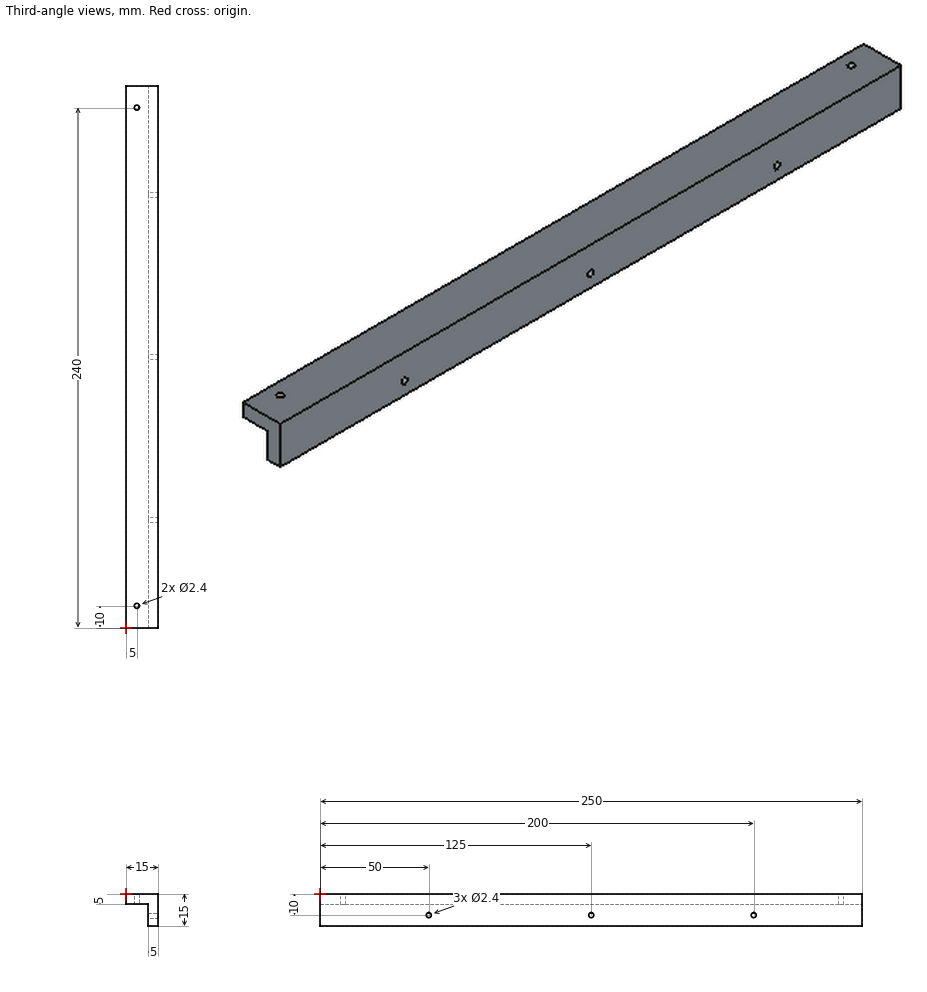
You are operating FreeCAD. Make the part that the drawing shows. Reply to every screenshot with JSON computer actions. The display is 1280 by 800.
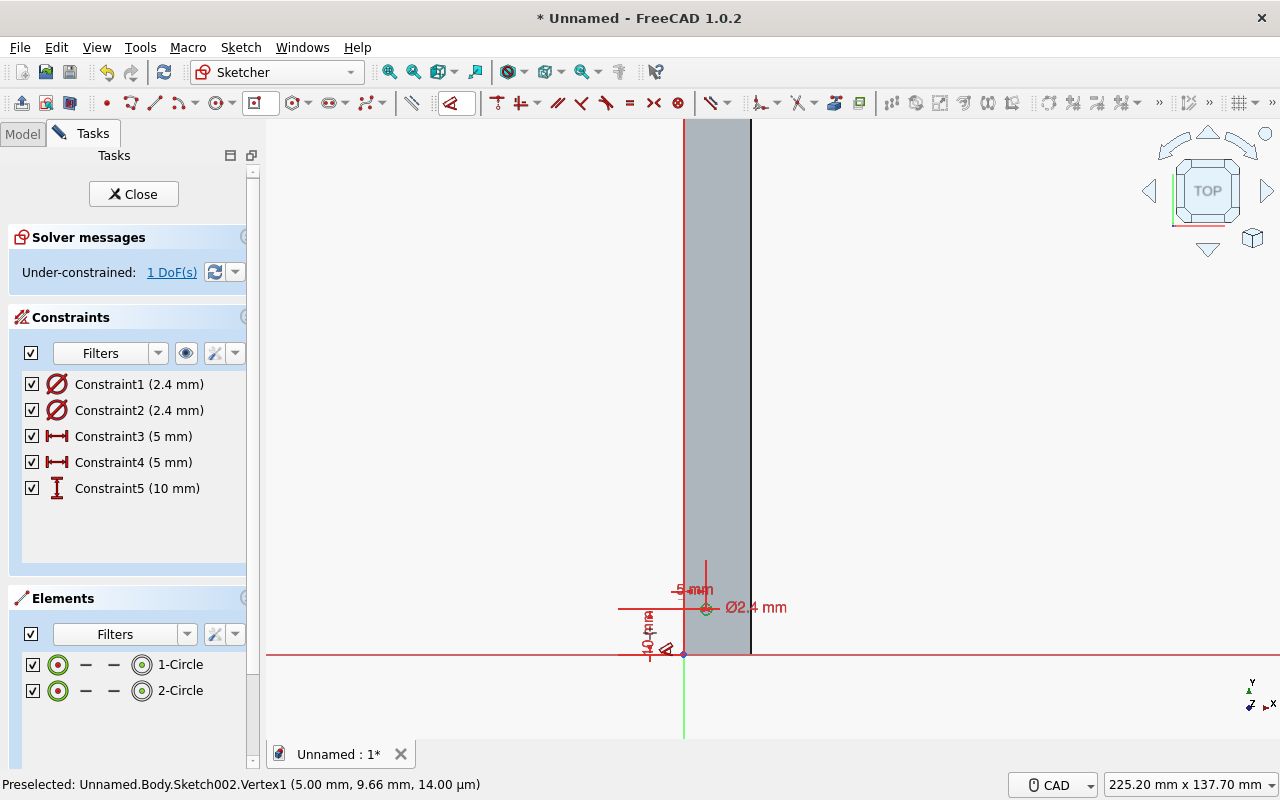
{"action": "scroll", "coordinate": [708, 614], "scroll_direction": "down", "scroll_amount": 5}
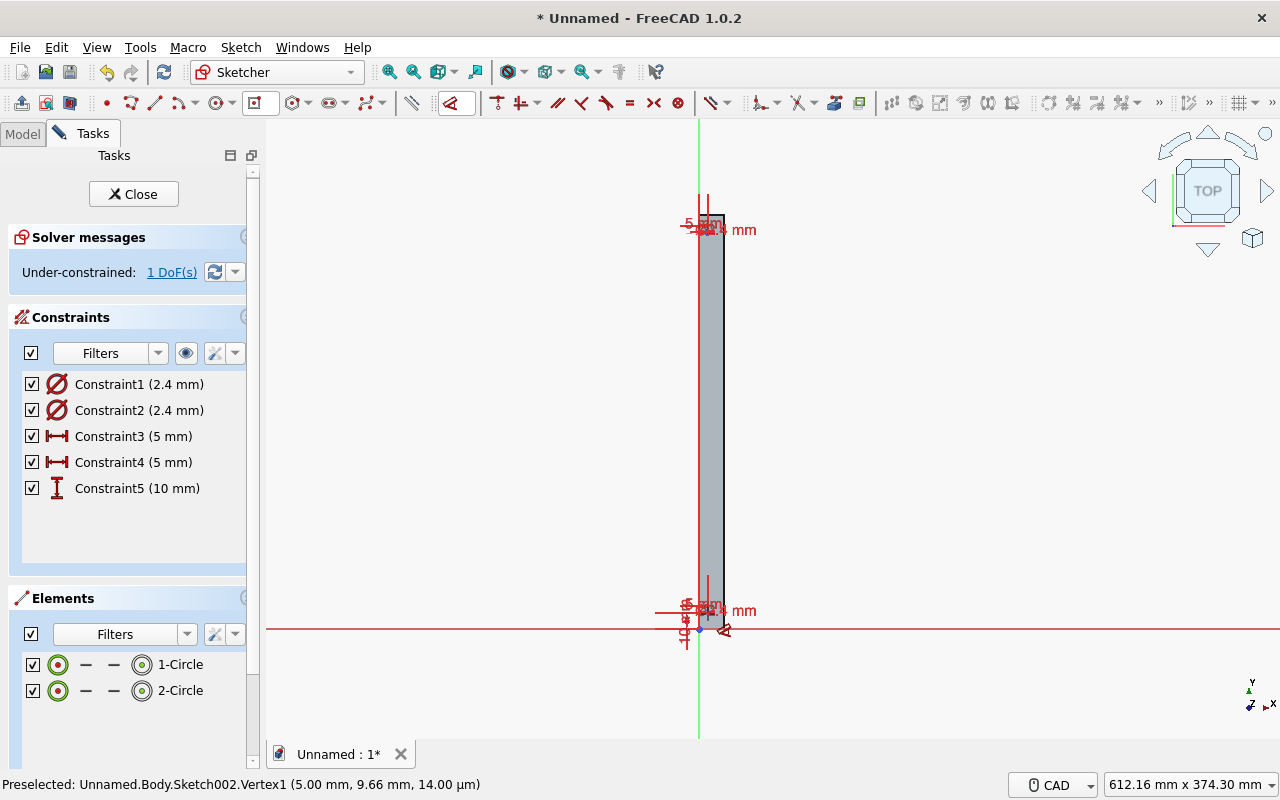
{"action": "left_click", "coordinate": [708, 232]}
{"action": "left_click", "coordinate": [665, 431]}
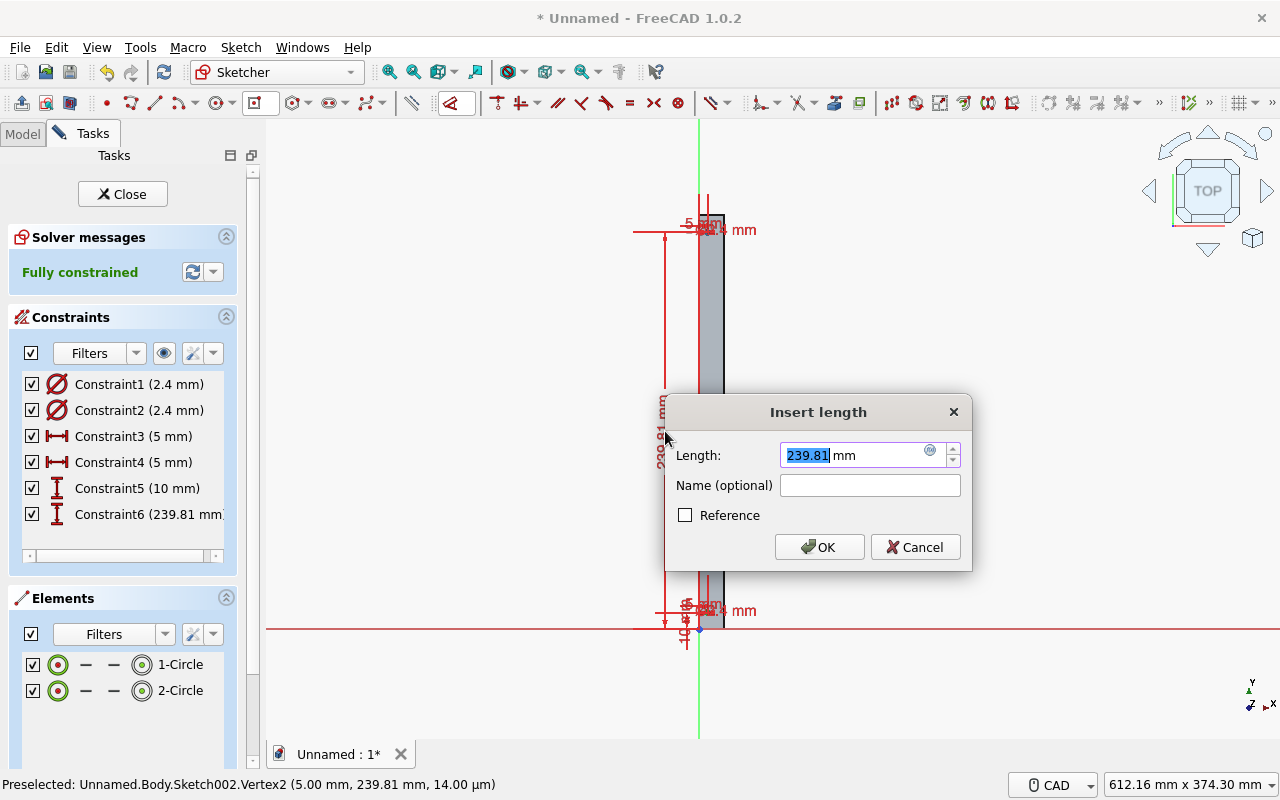
{"action": "type", "text": "240"}
{"action": "key", "text": "Return"}
{"action": "key", "text": "Escape"}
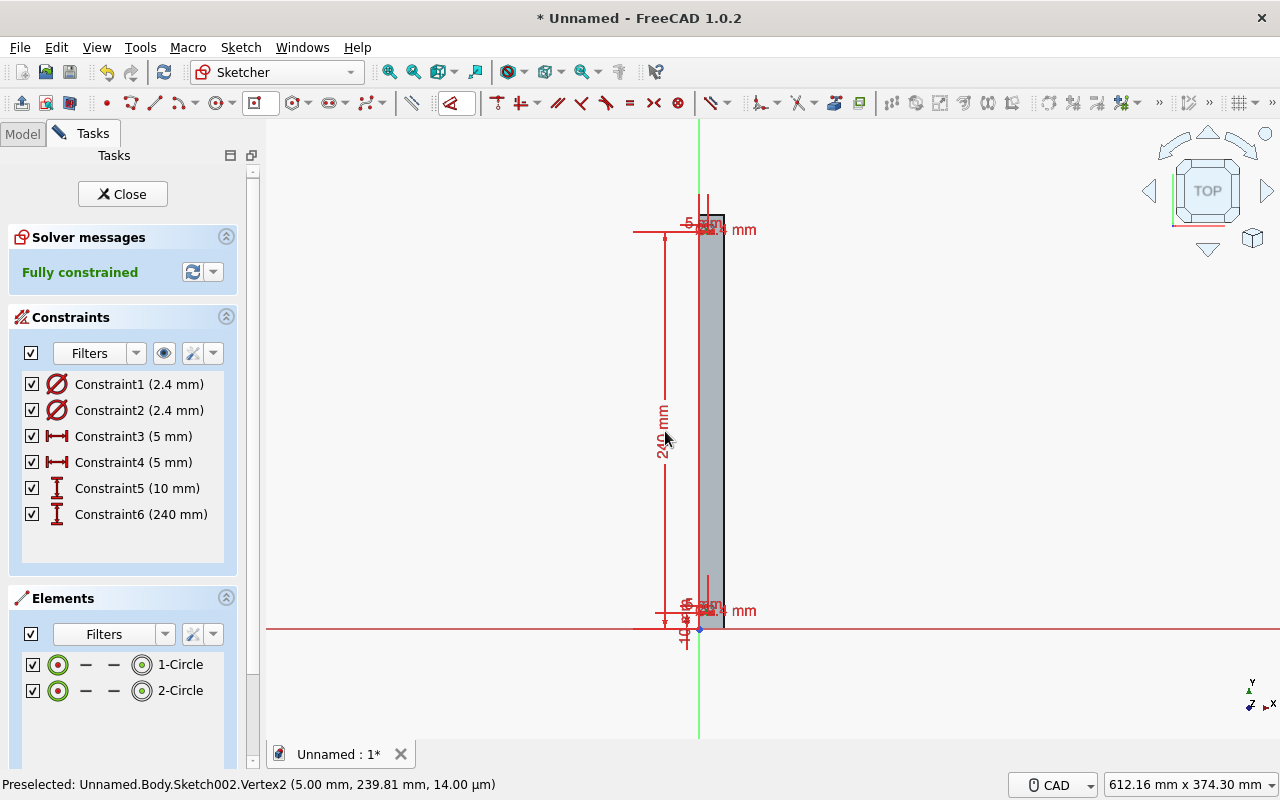
{"action": "left_click", "coordinate": [123, 194]}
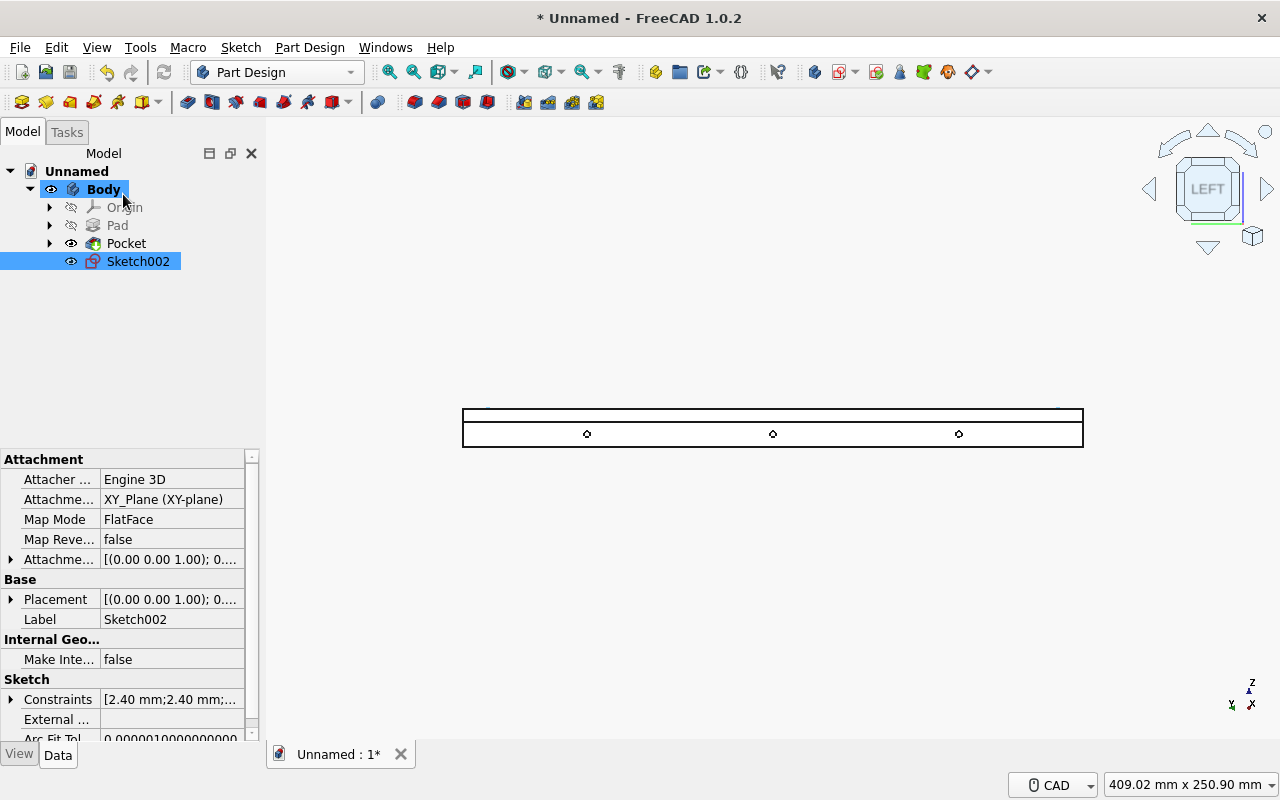
{"action": "left_click", "coordinate": [188, 102]}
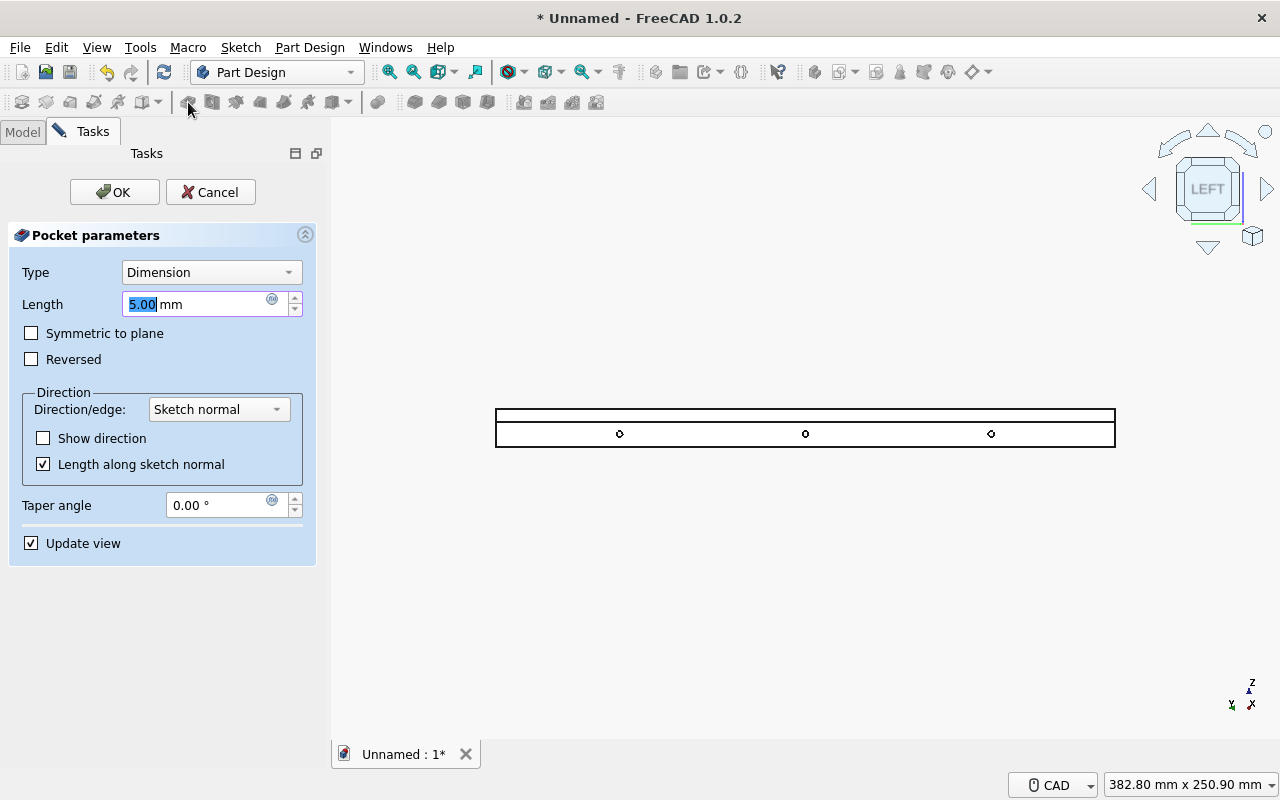
{"action": "type", "text": "5"}
{"action": "key", "text": "Tab"}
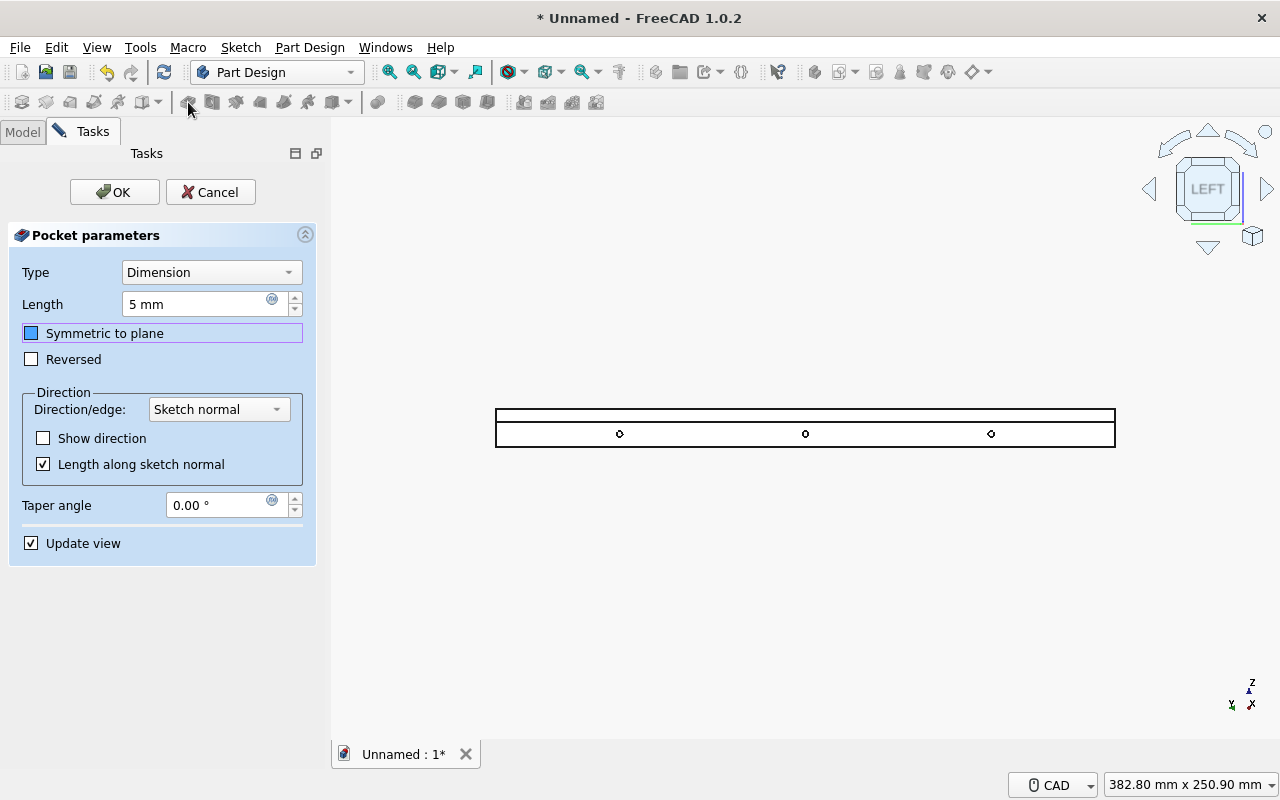
{"action": "left_click", "coordinate": [115, 192]}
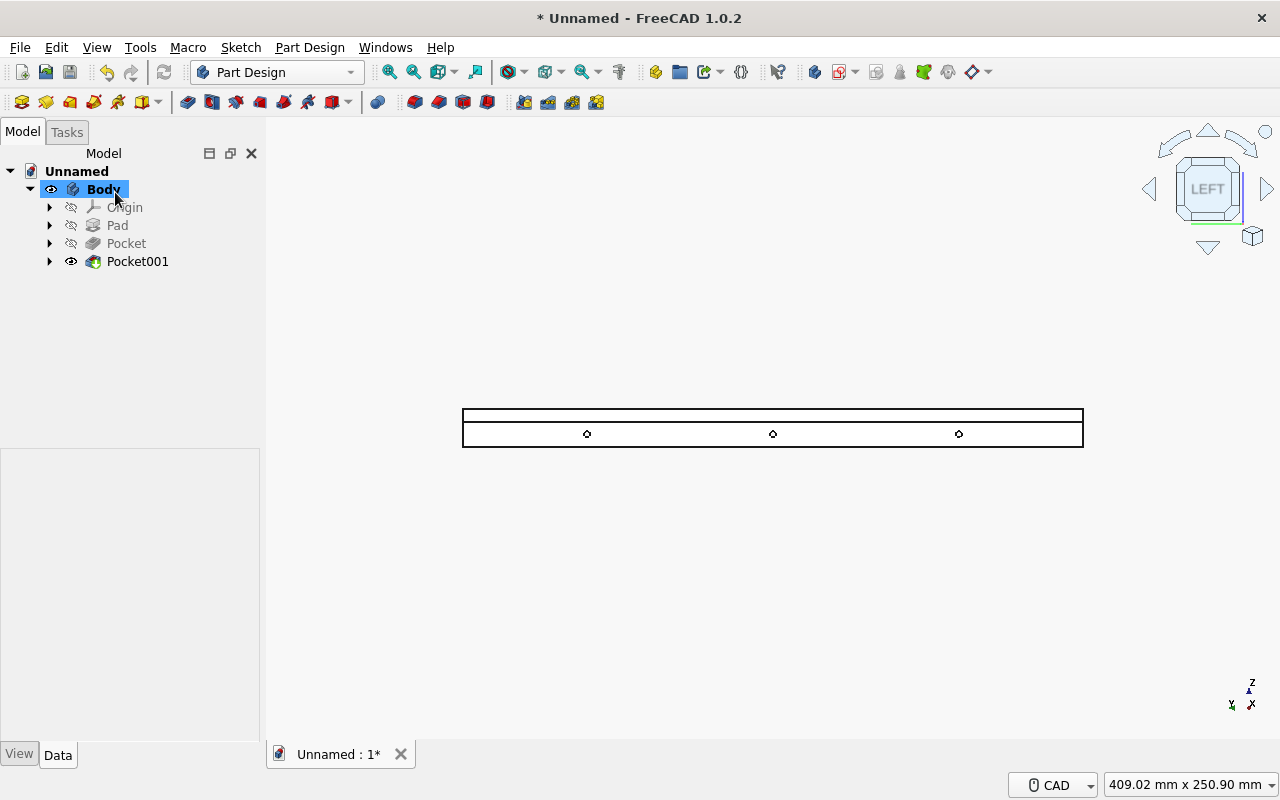
{"action": "key", "text": "0"}